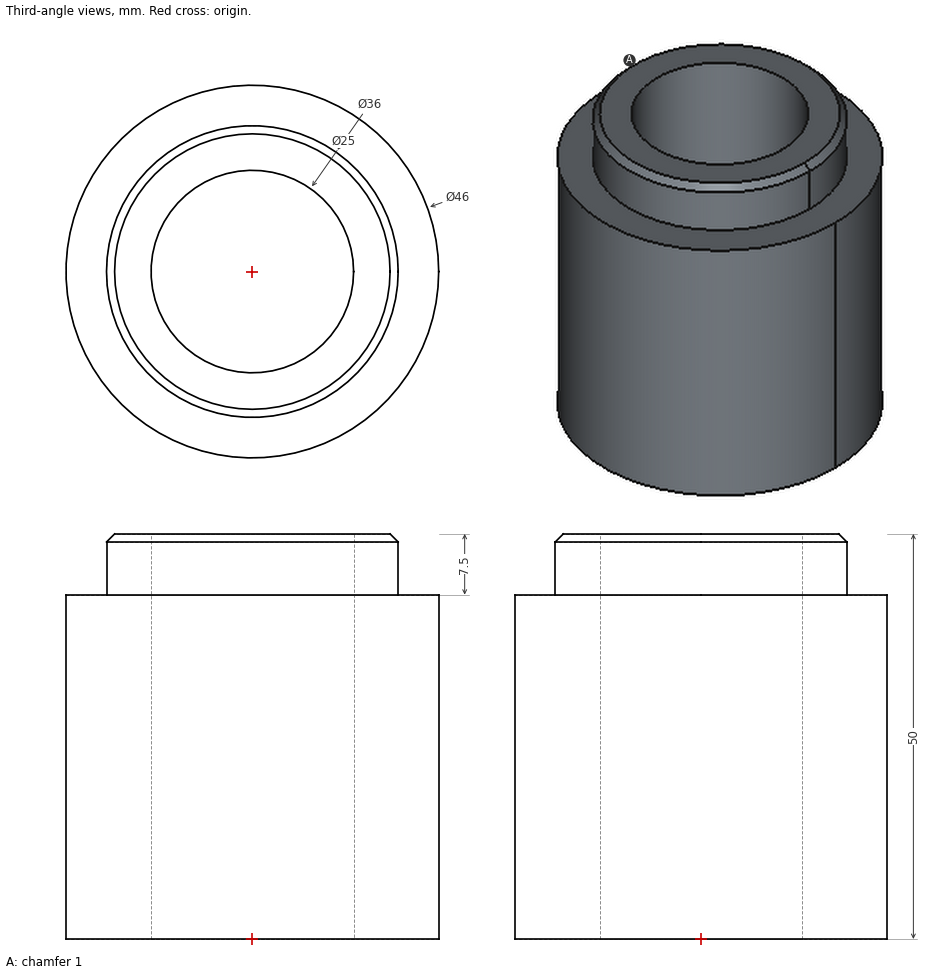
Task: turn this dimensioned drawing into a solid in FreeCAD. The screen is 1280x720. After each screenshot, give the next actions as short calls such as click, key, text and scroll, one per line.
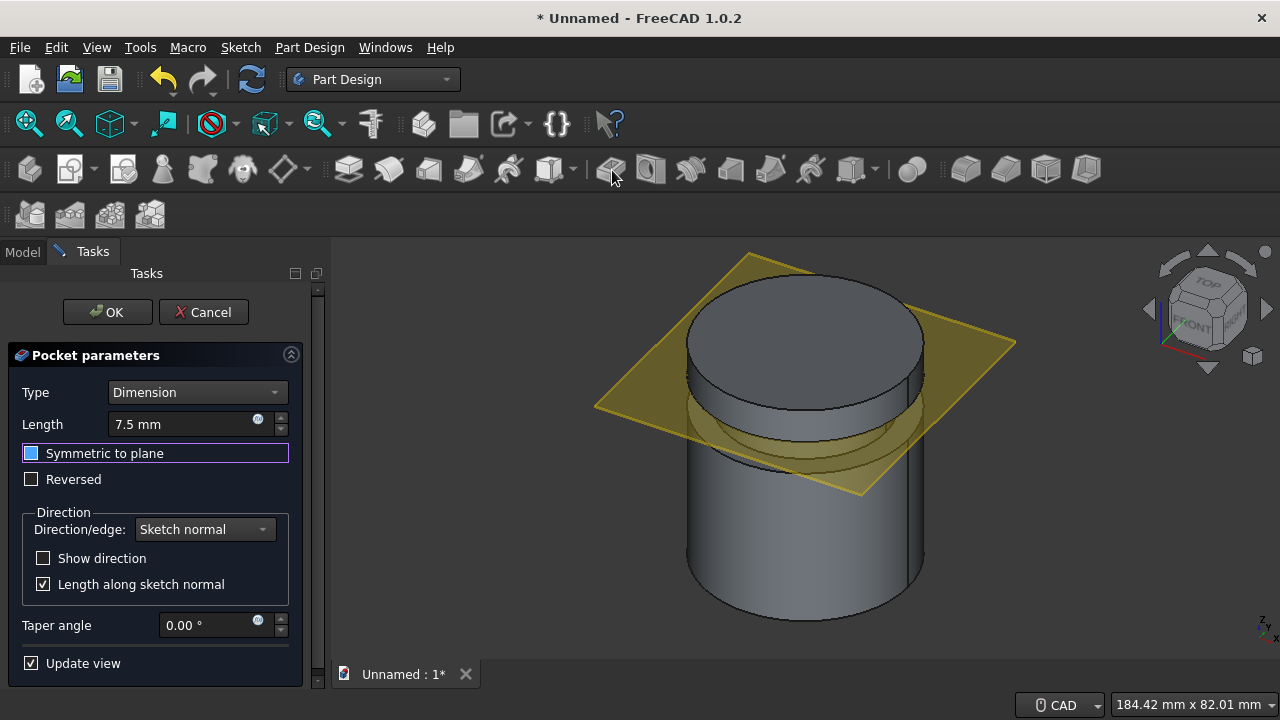
click(30, 479)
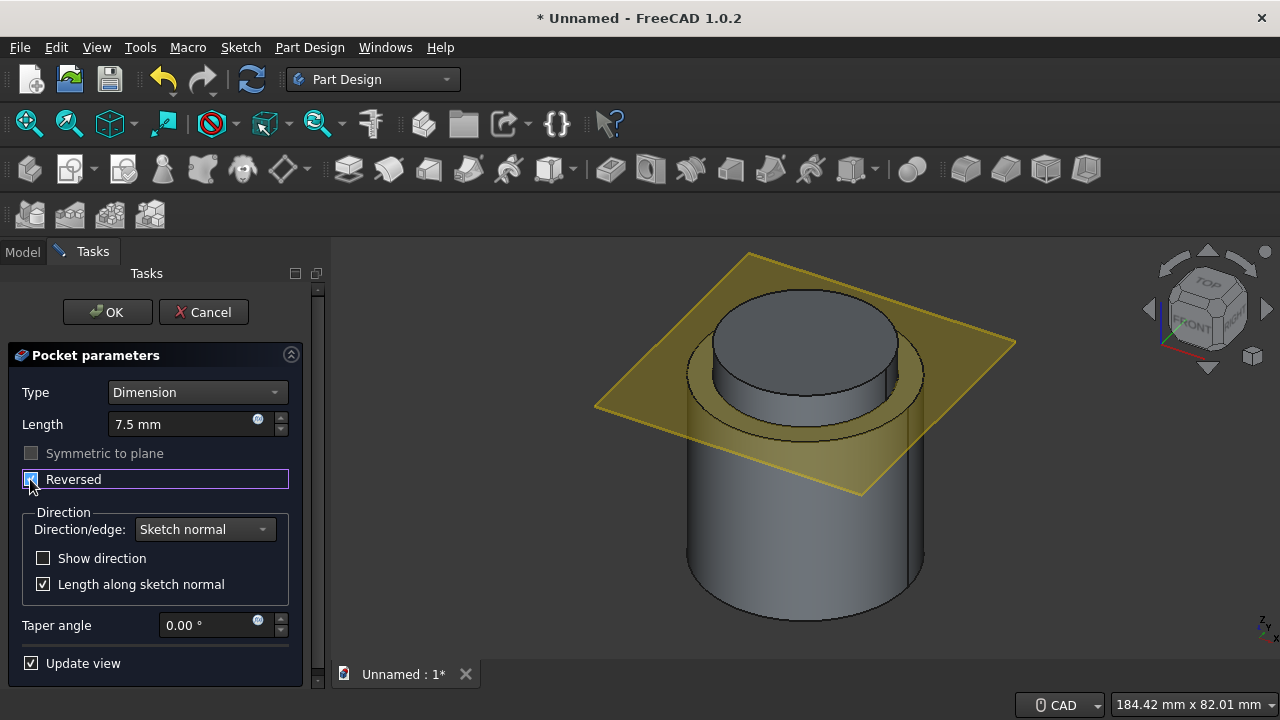
click(108, 312)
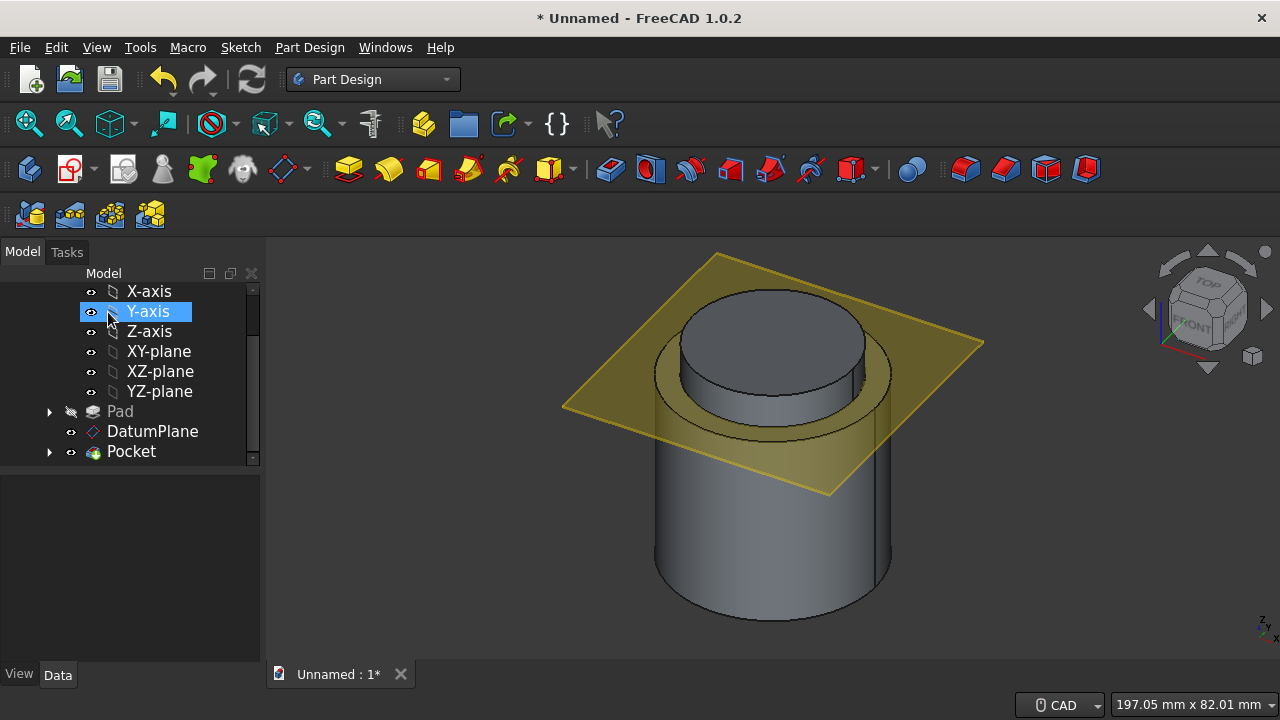
click(116, 432)
key(space)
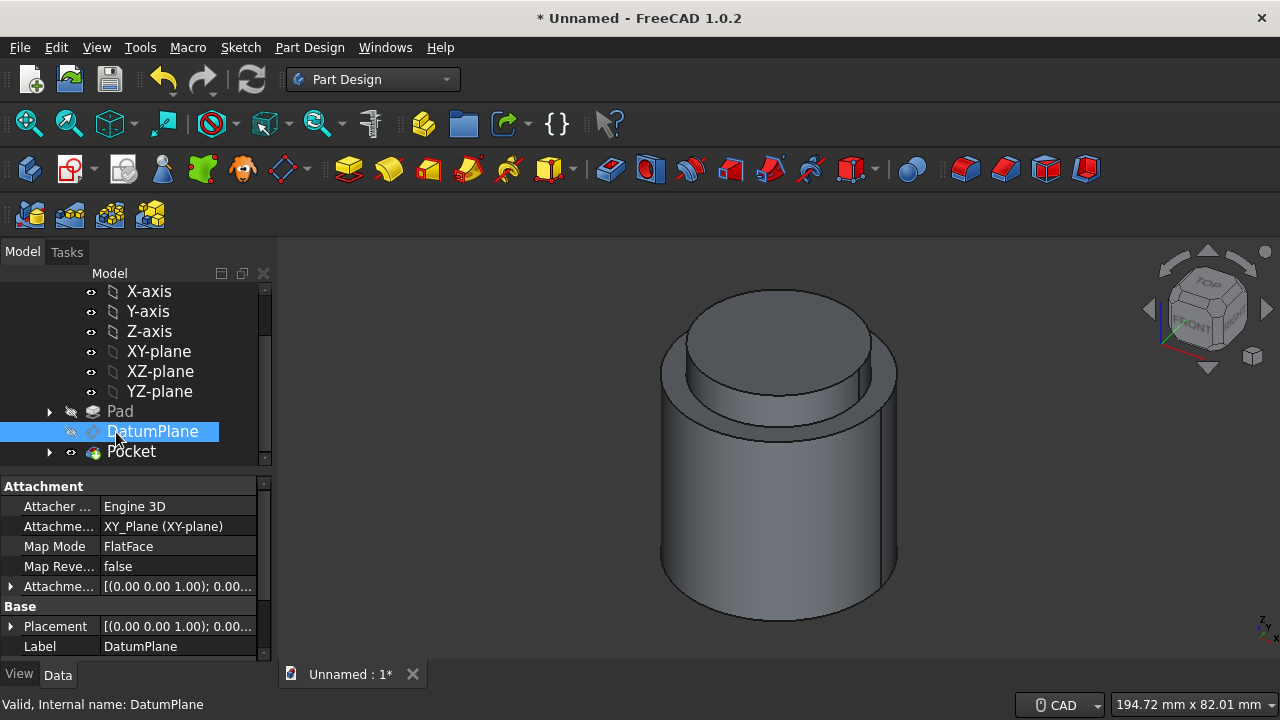
click(779, 342)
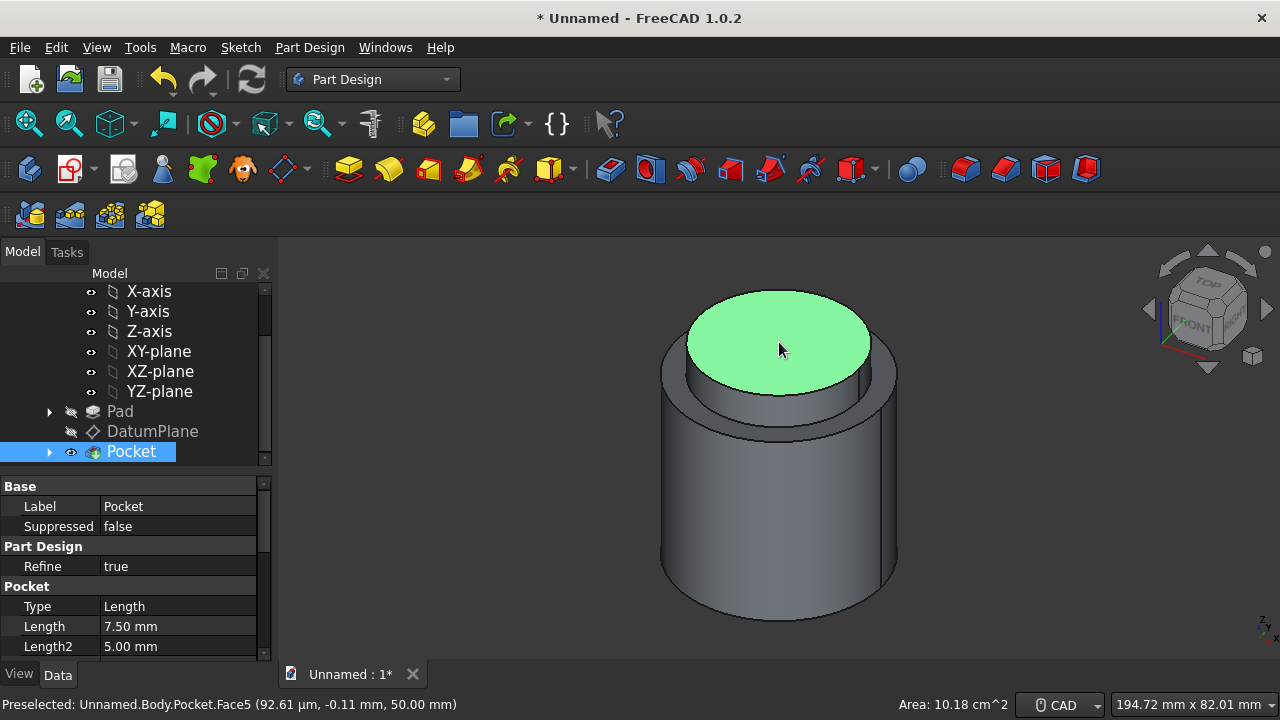
click(70, 170)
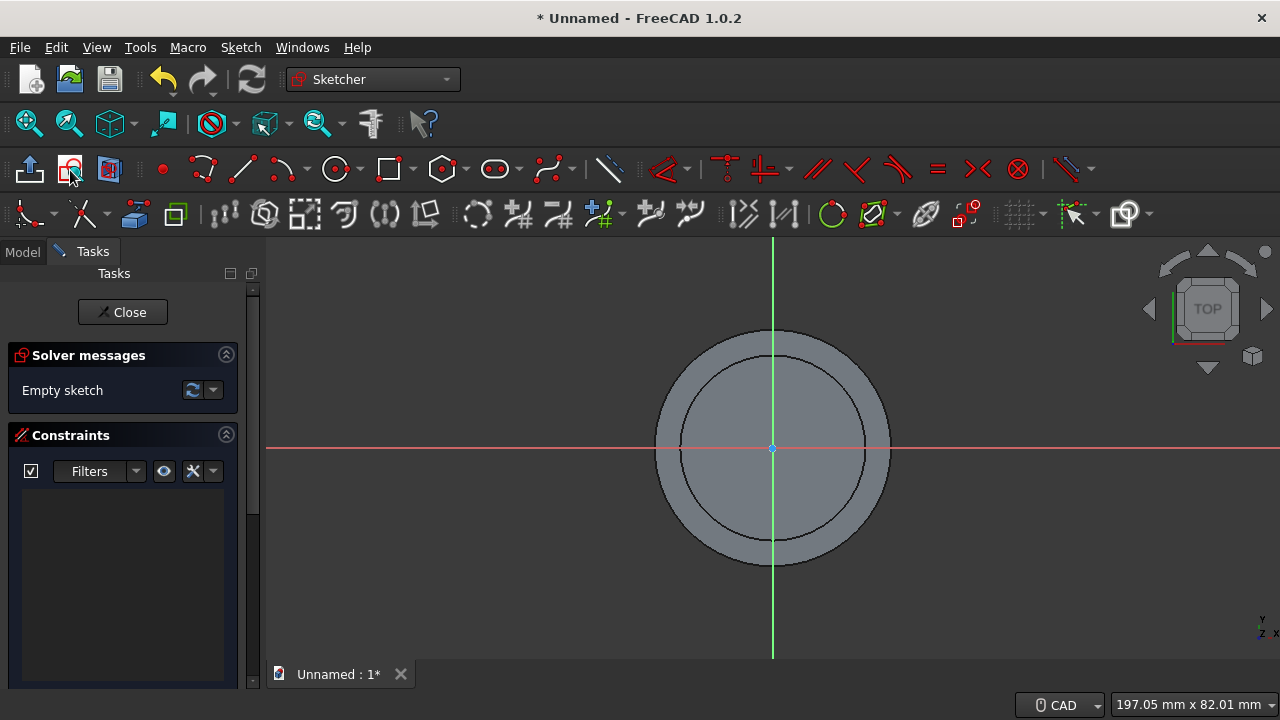
scroll(856, 448, up, 3)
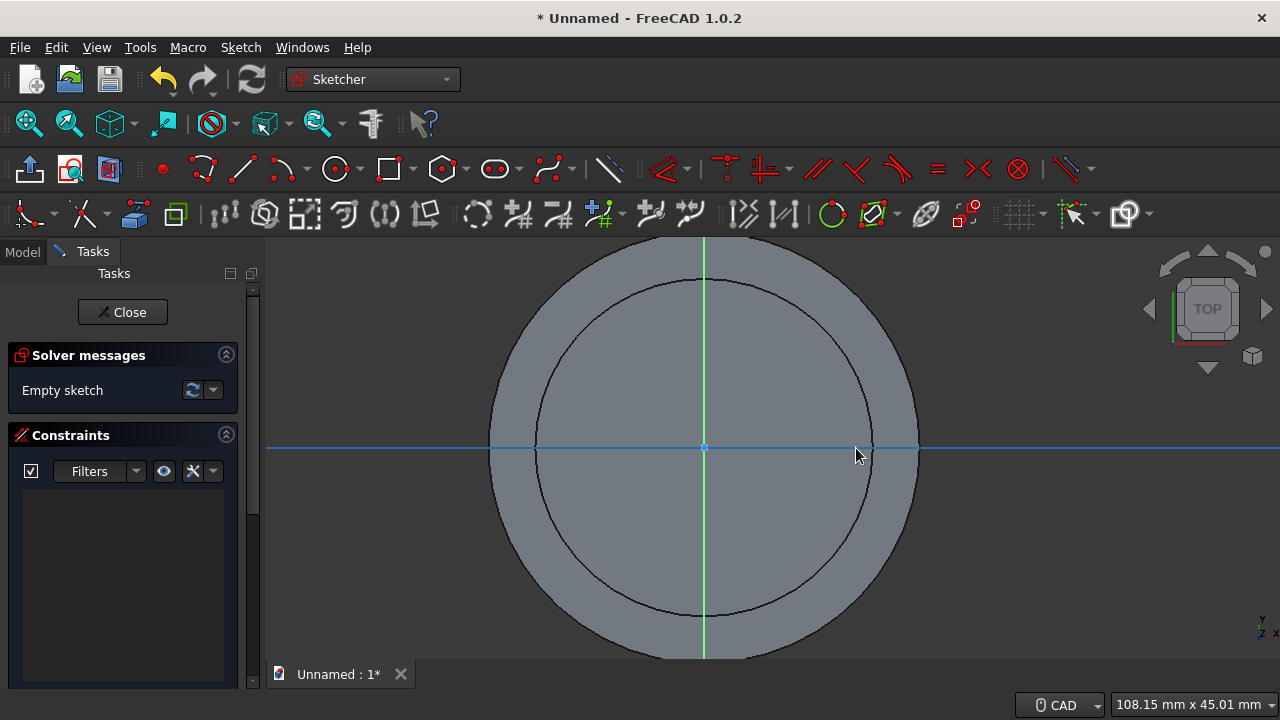
key(g)
key(c)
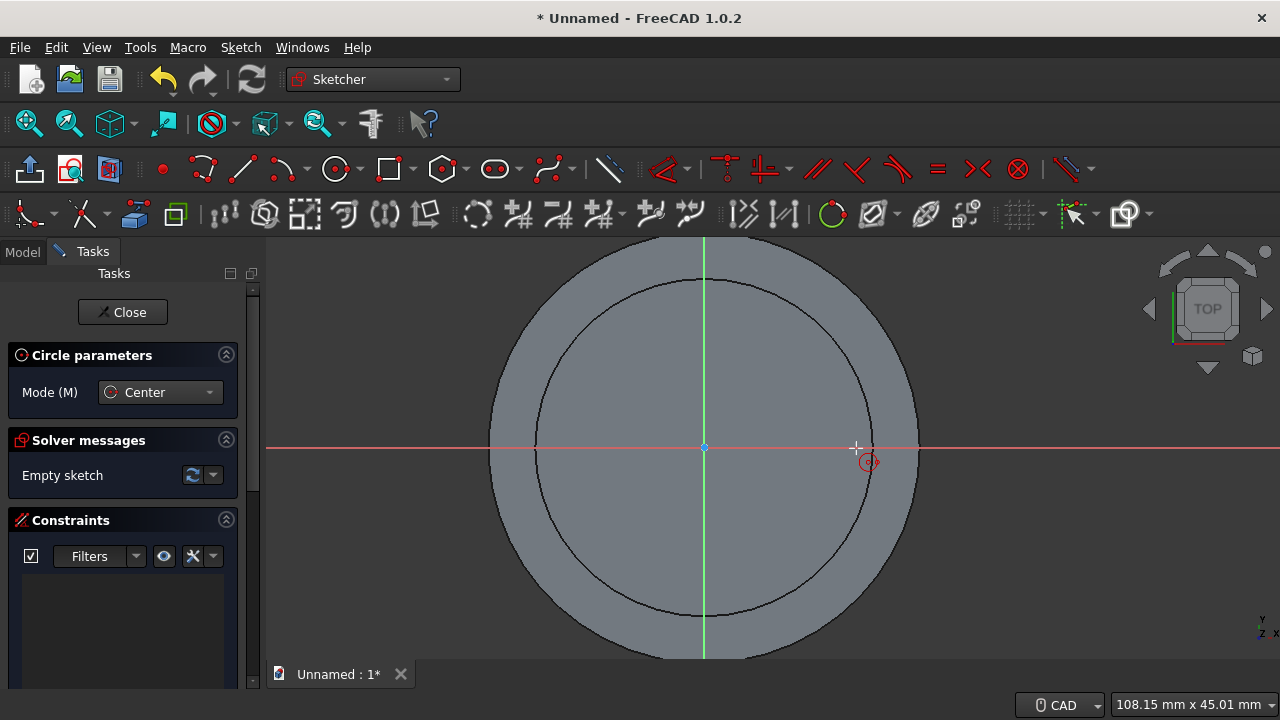
click(704, 448)
move(787, 365)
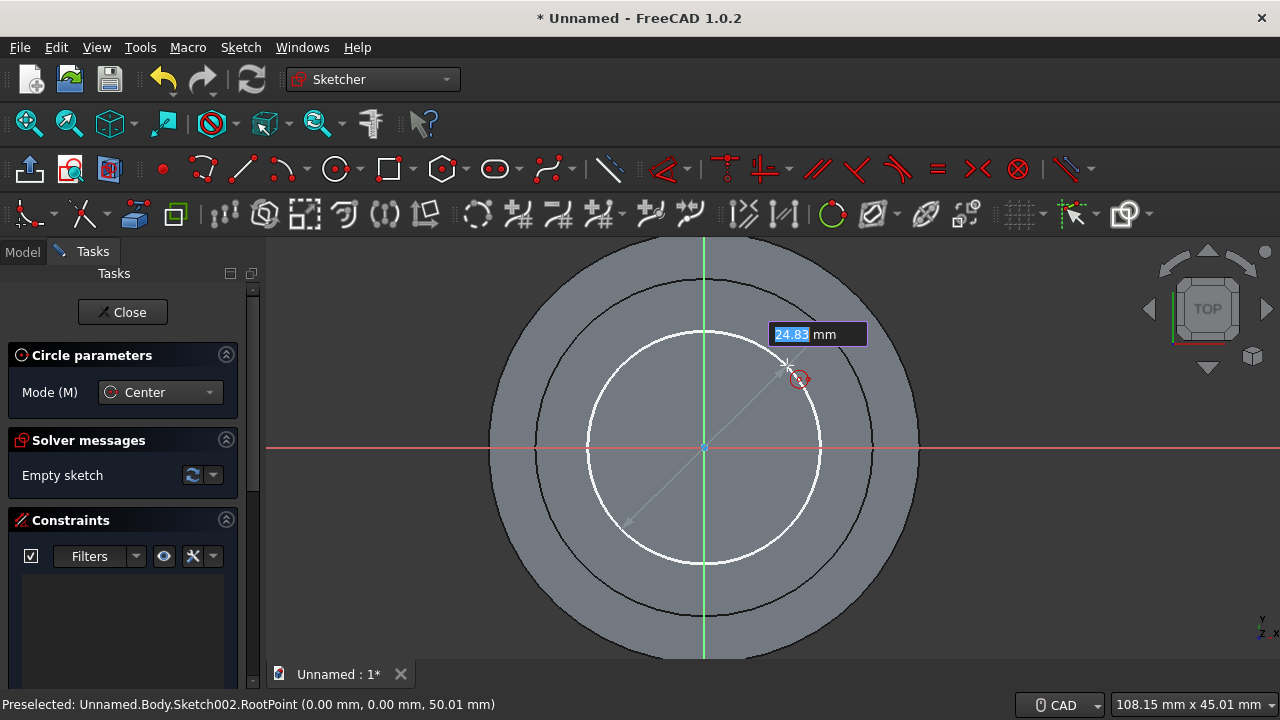
text(25)
key(Return)
key(Escape)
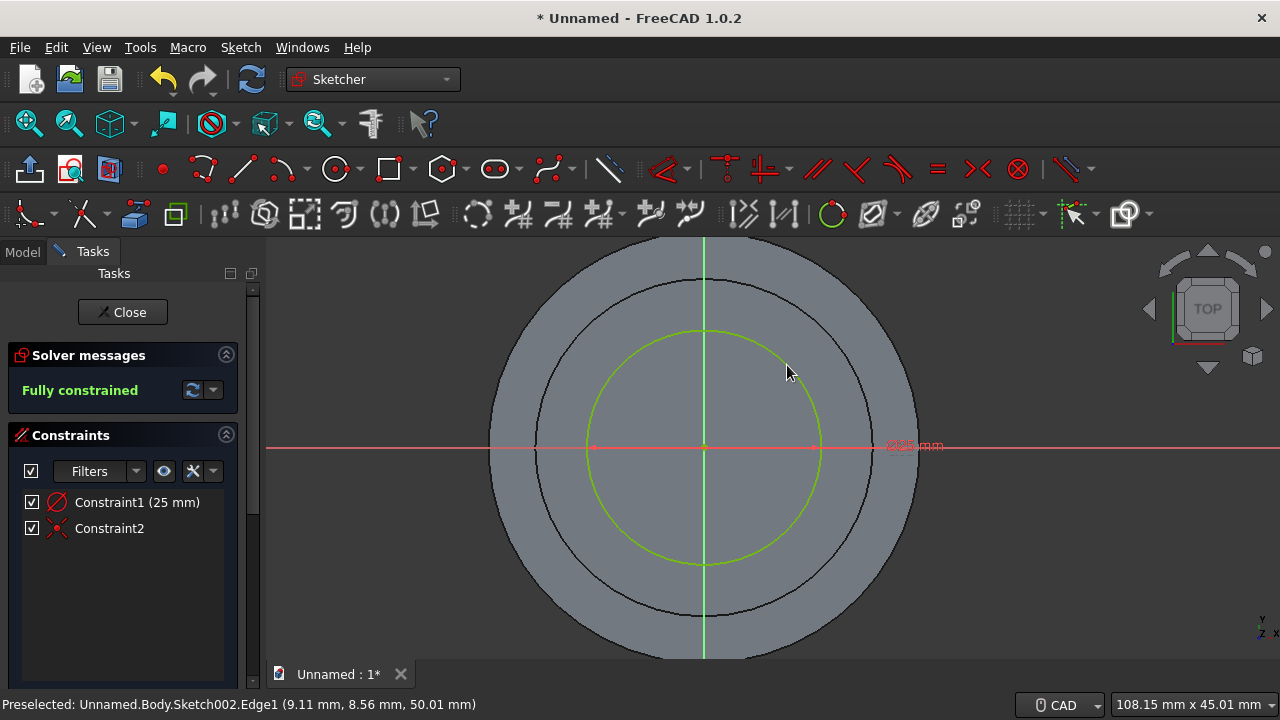
click(123, 312)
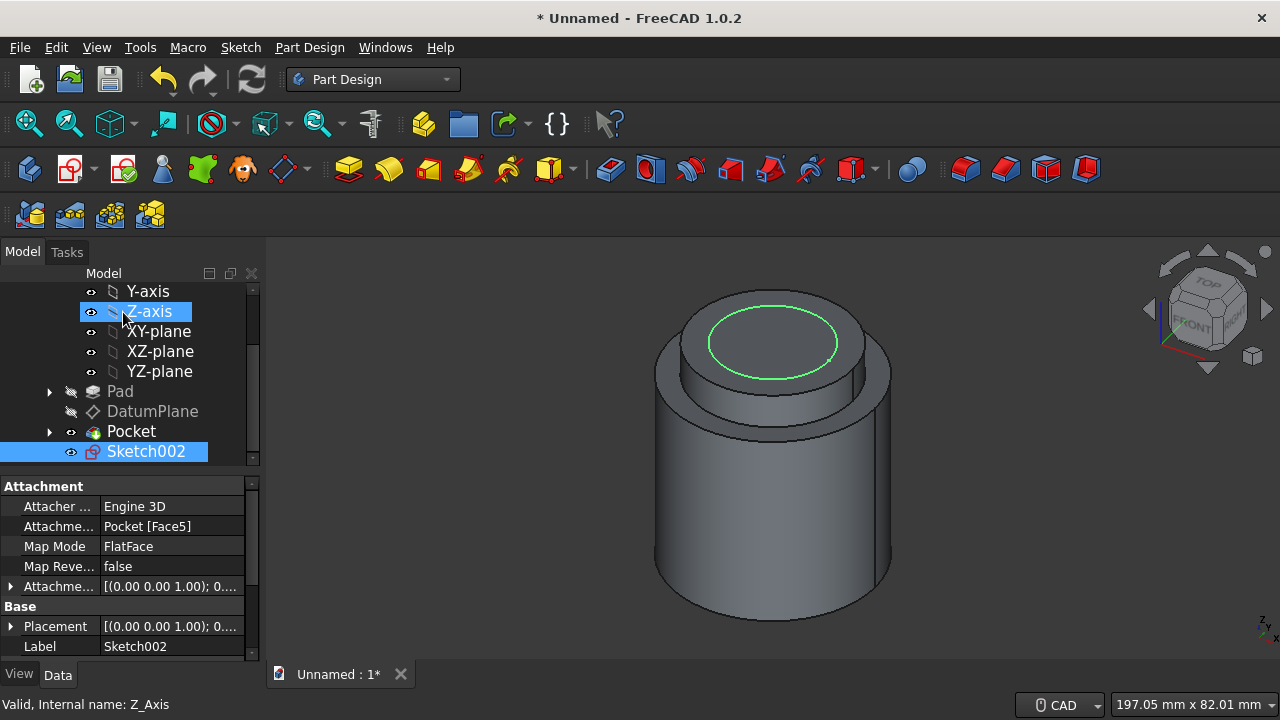
click(612, 170)